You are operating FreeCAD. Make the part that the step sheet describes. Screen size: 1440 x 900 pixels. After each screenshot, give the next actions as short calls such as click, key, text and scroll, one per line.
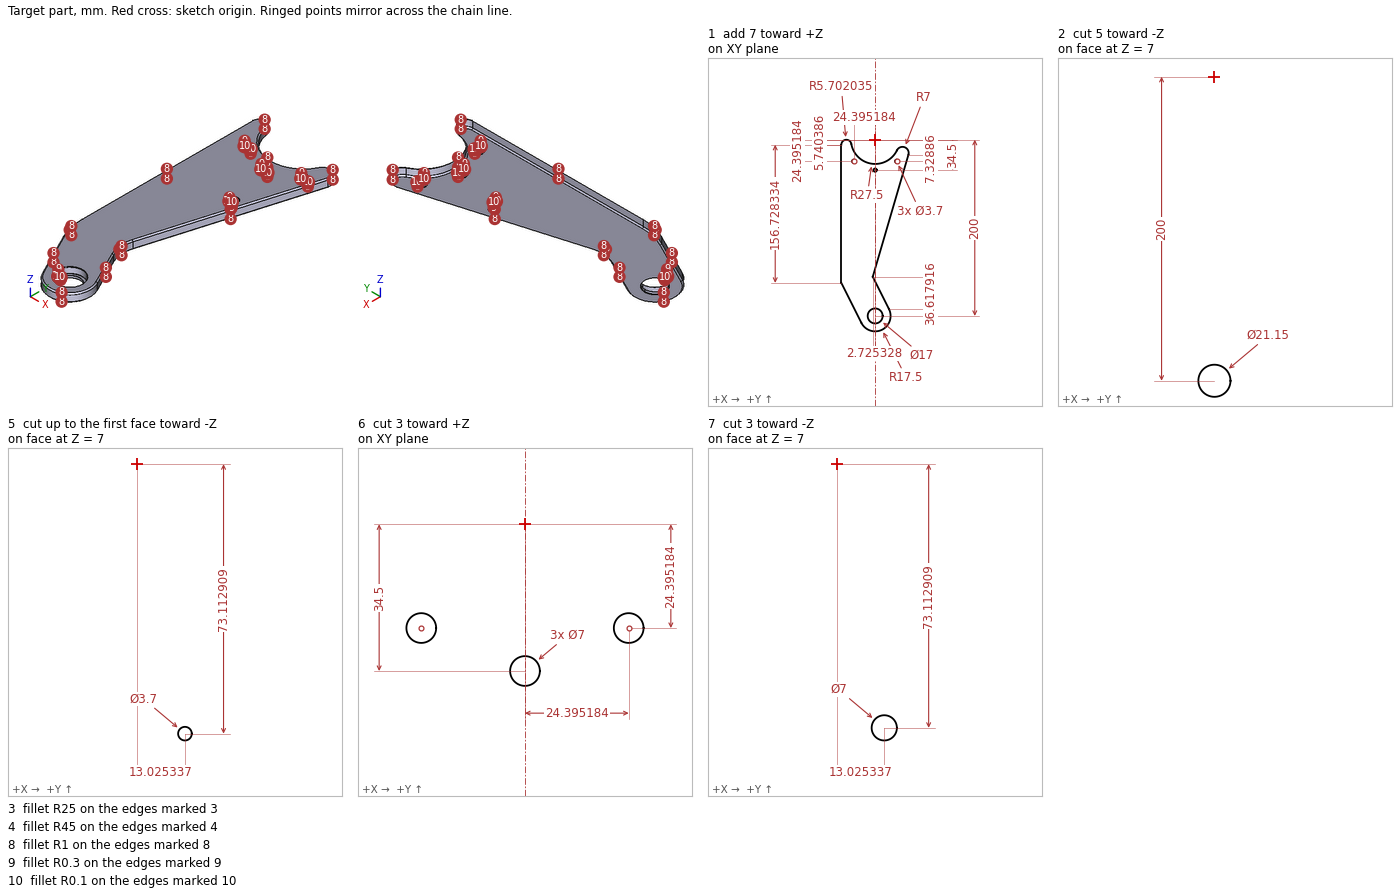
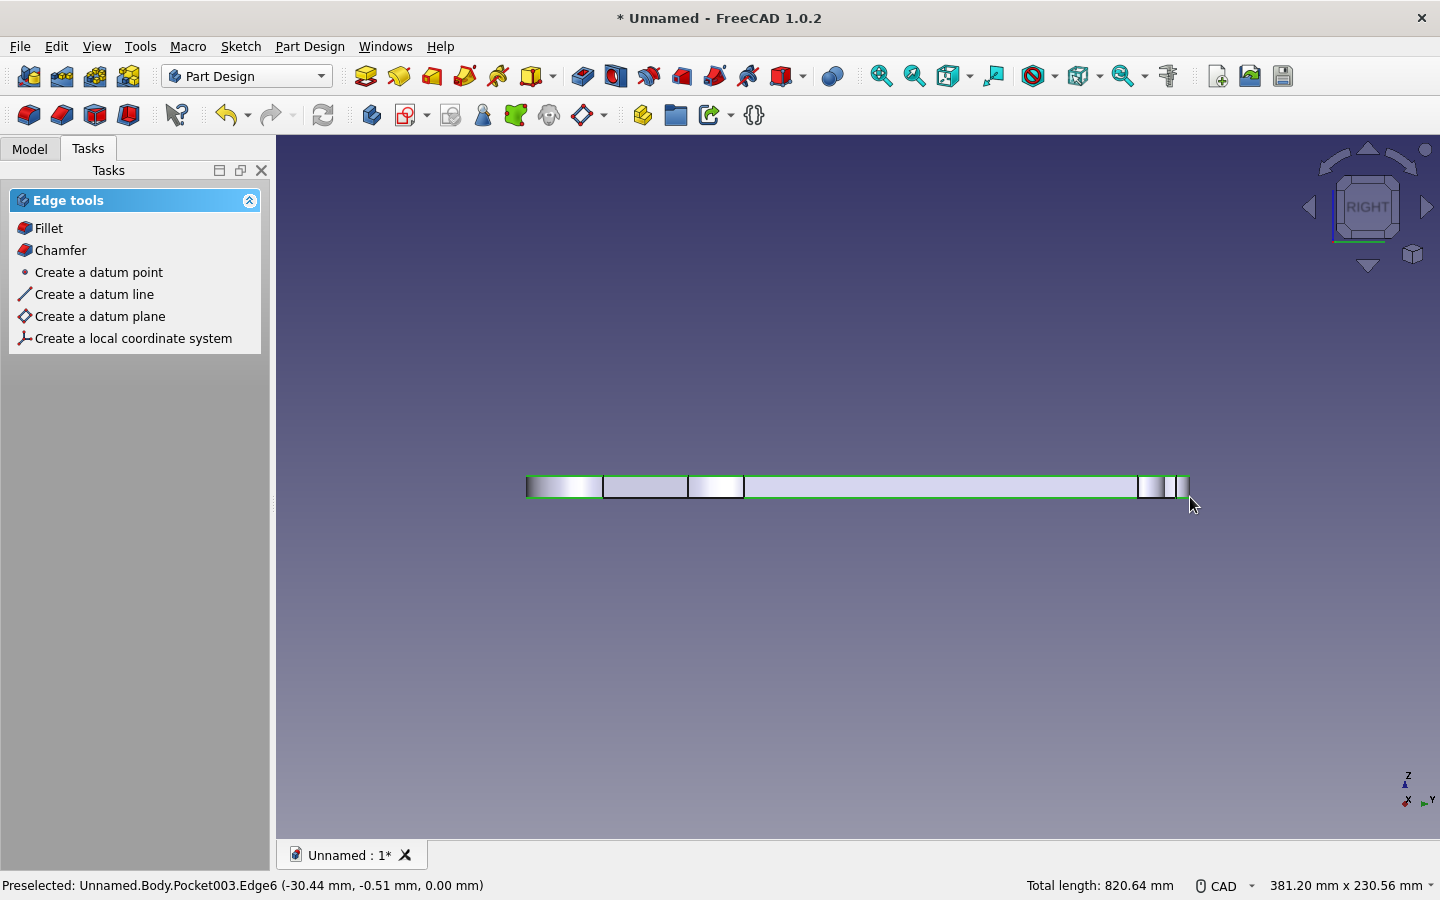
click(1169, 497, ctrl)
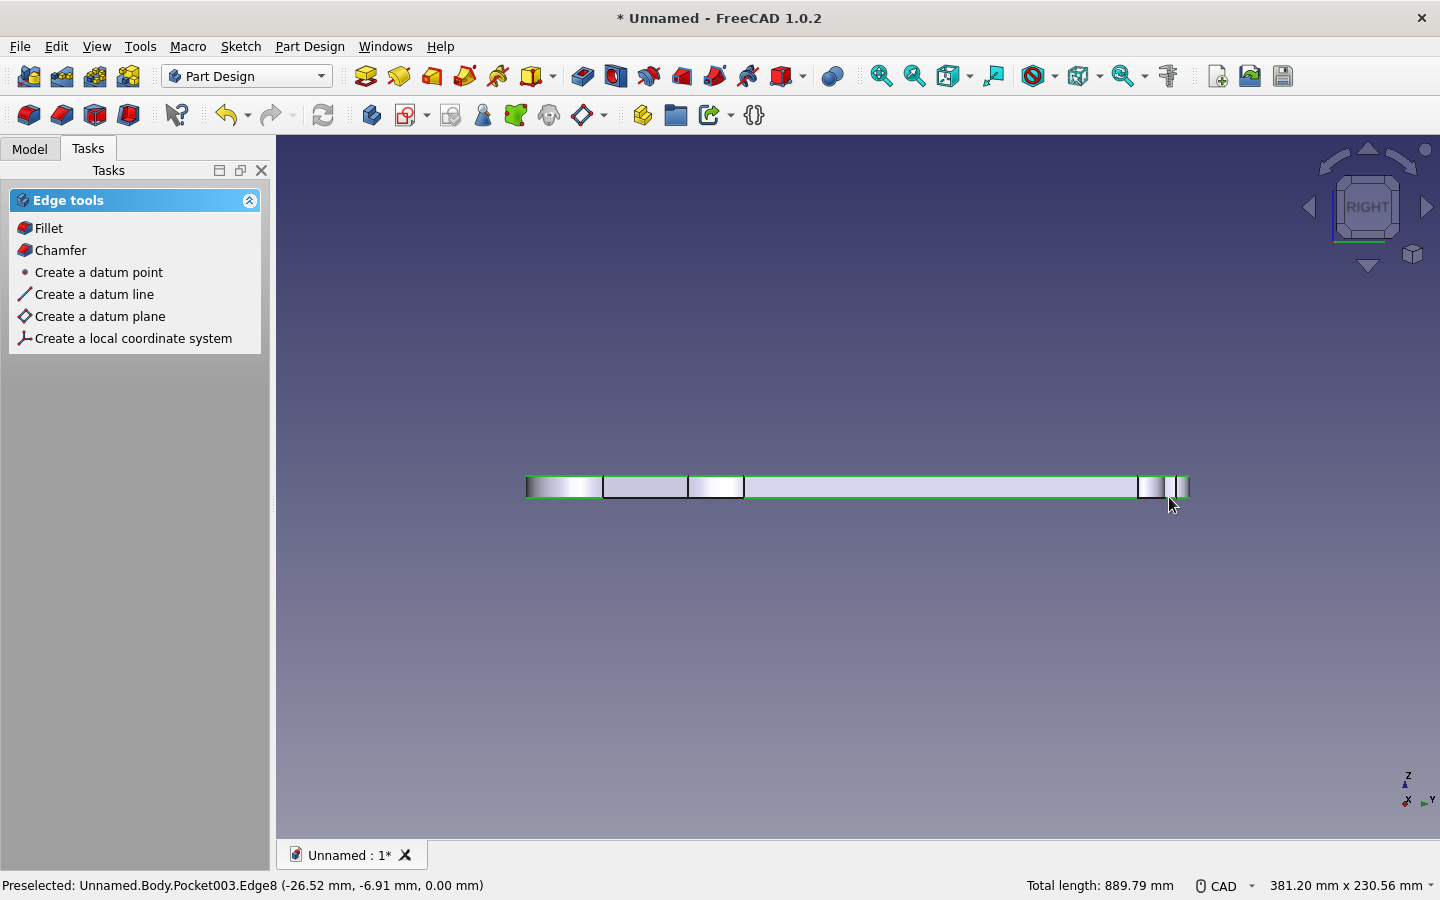
click(1164, 497, ctrl)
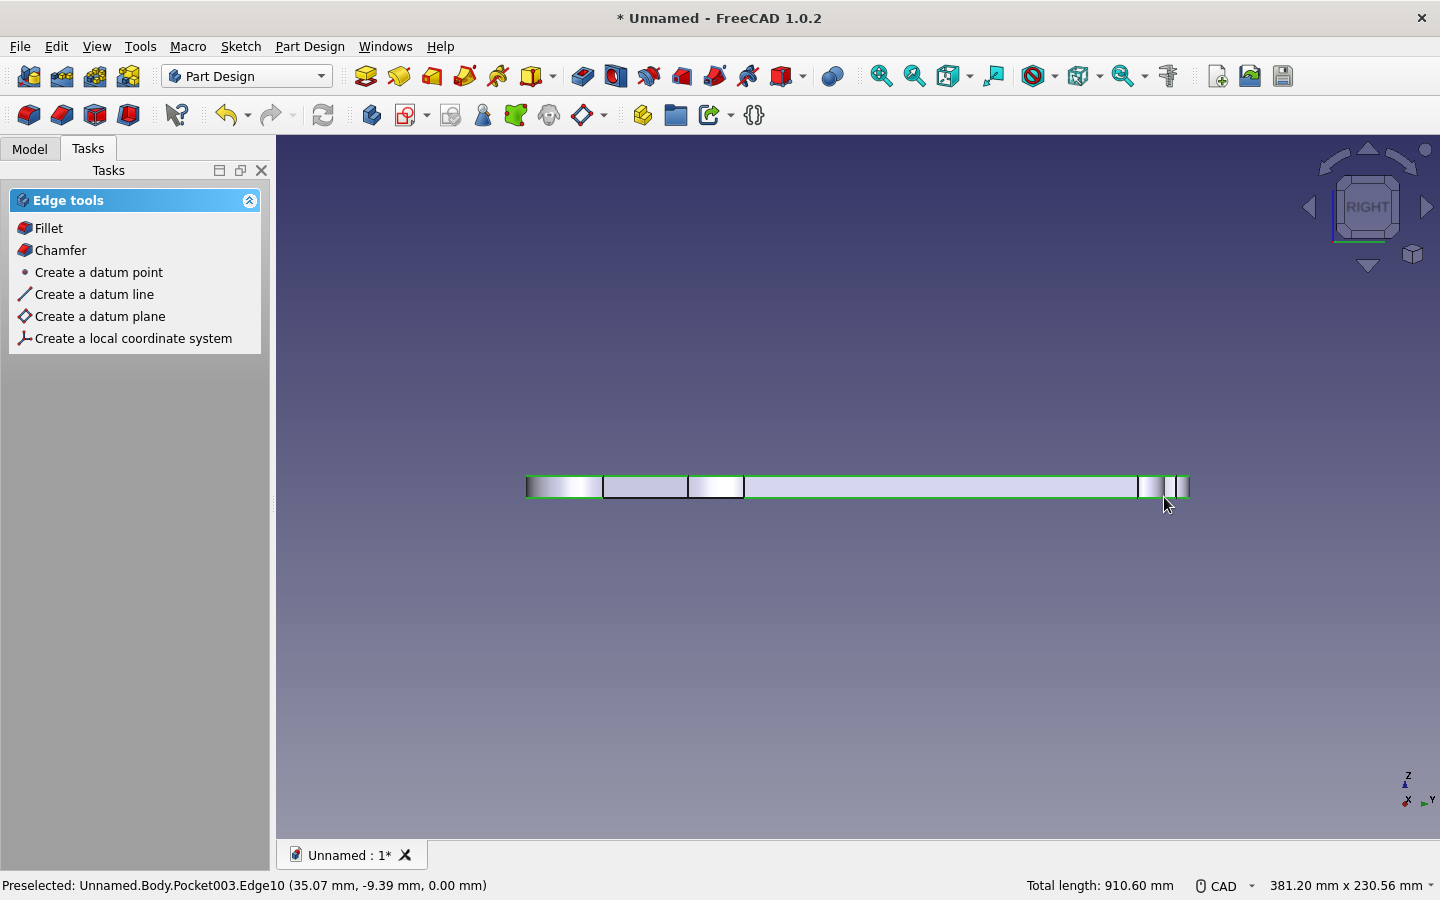
click(646, 497, ctrl)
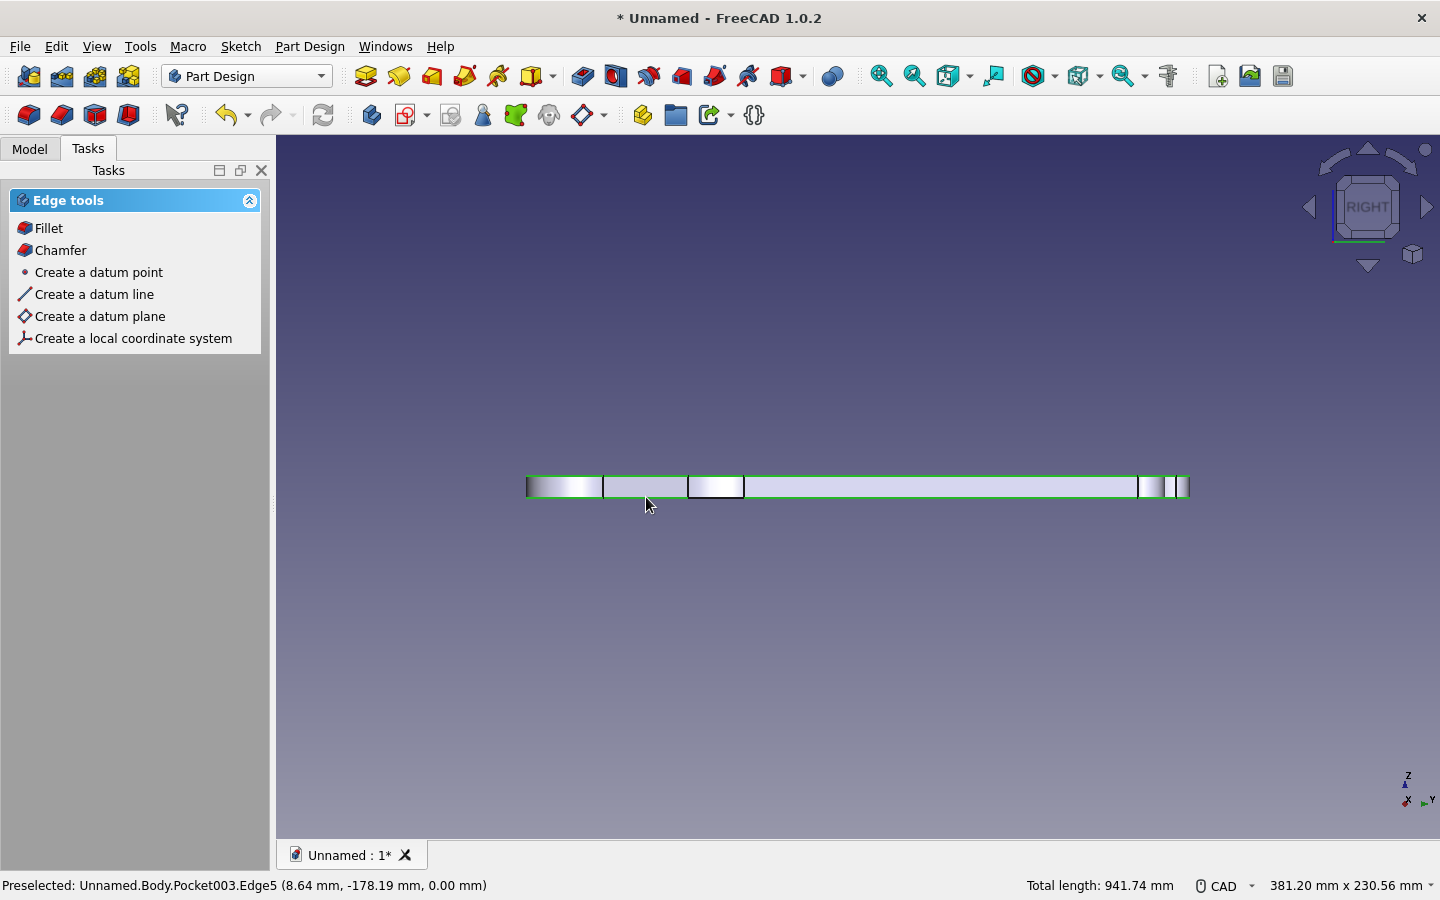
click(716, 497, ctrl)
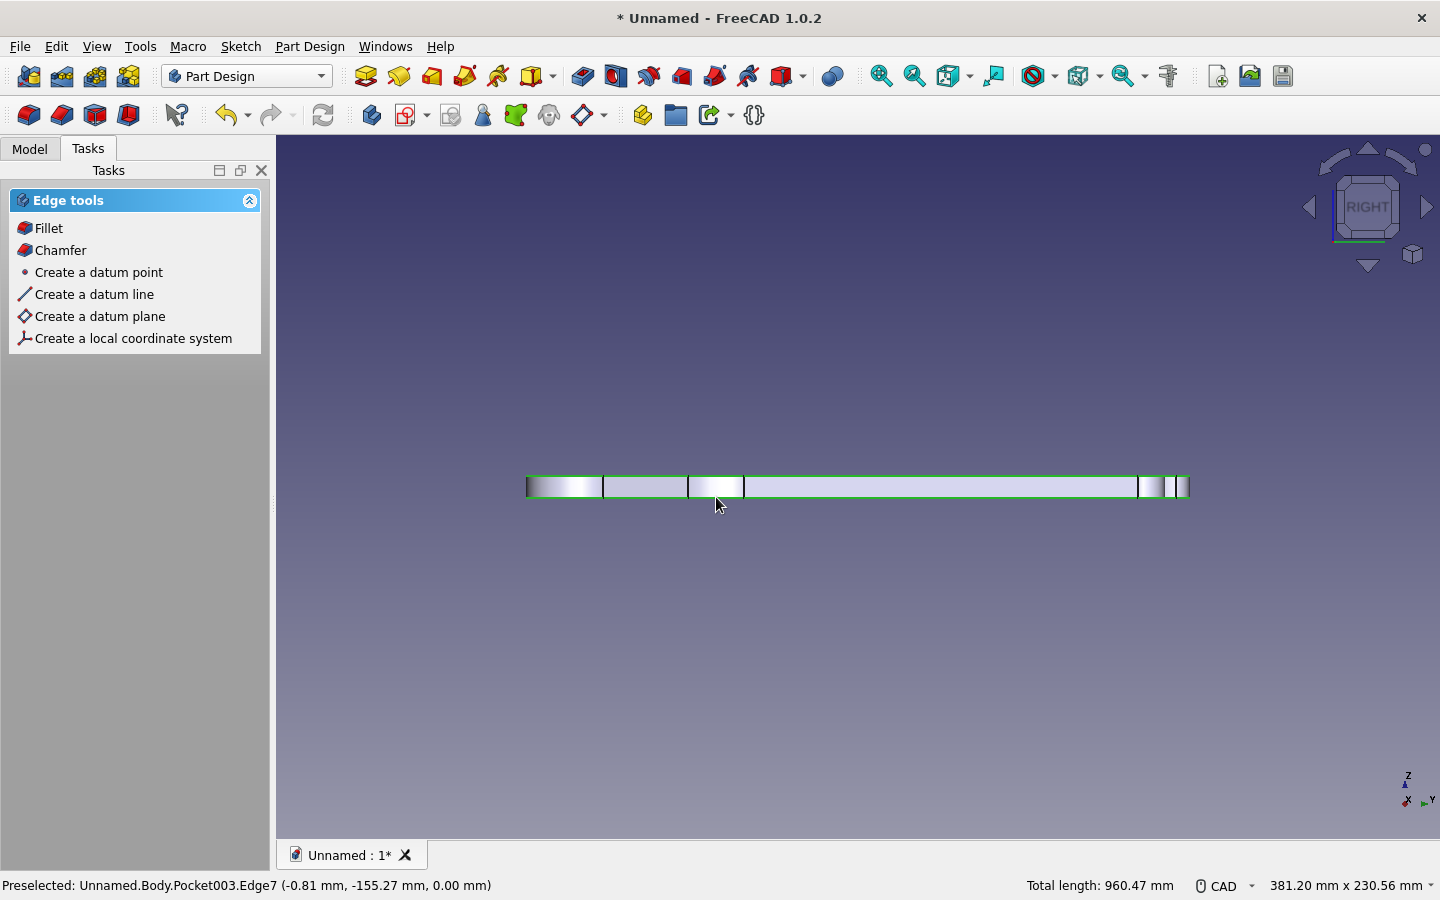
key(5)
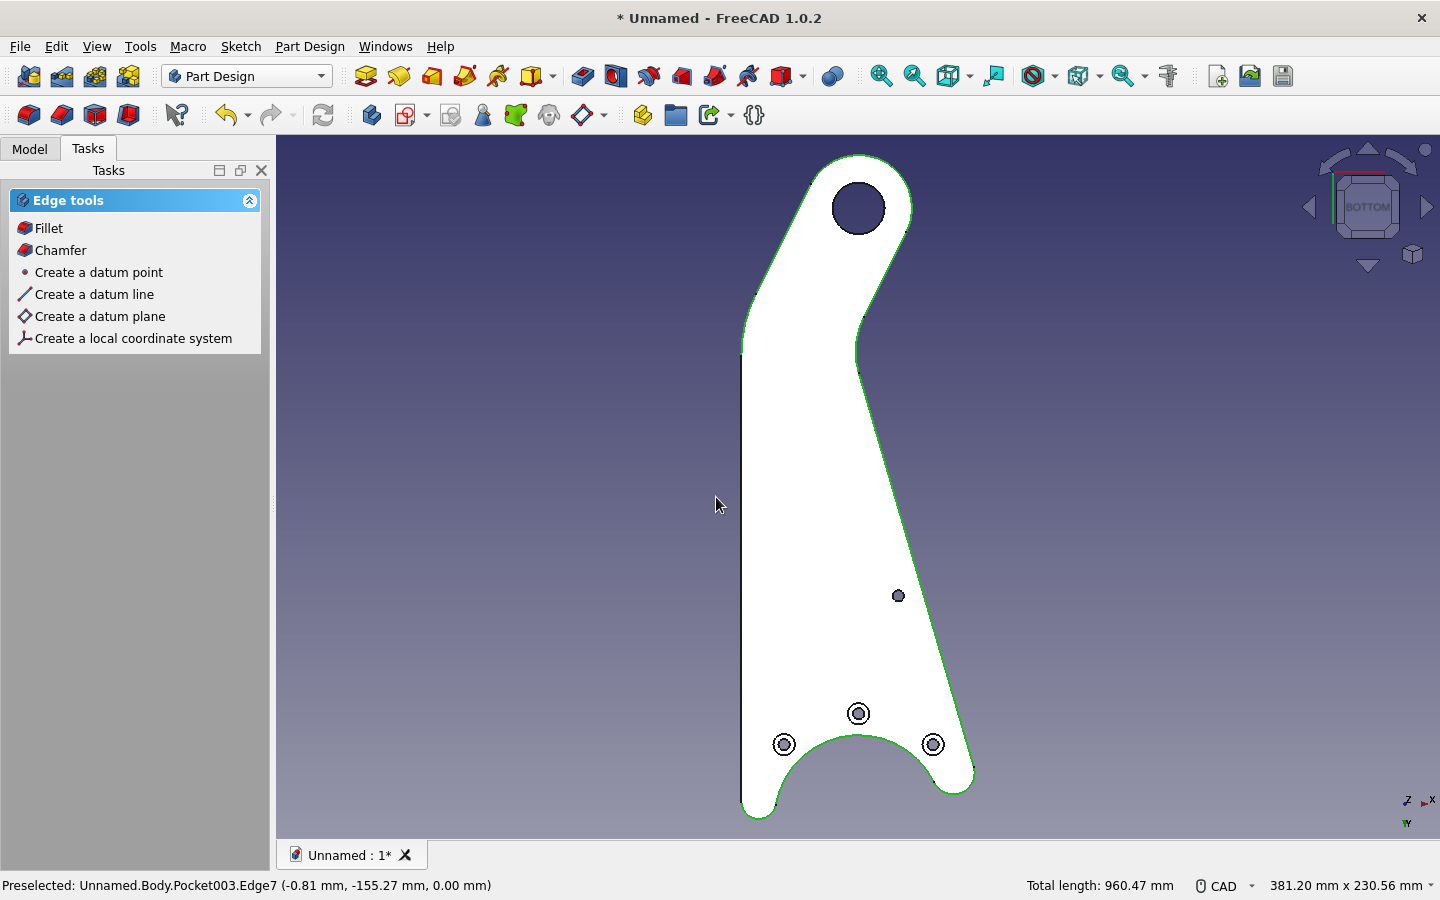
click(741, 578, ctrl)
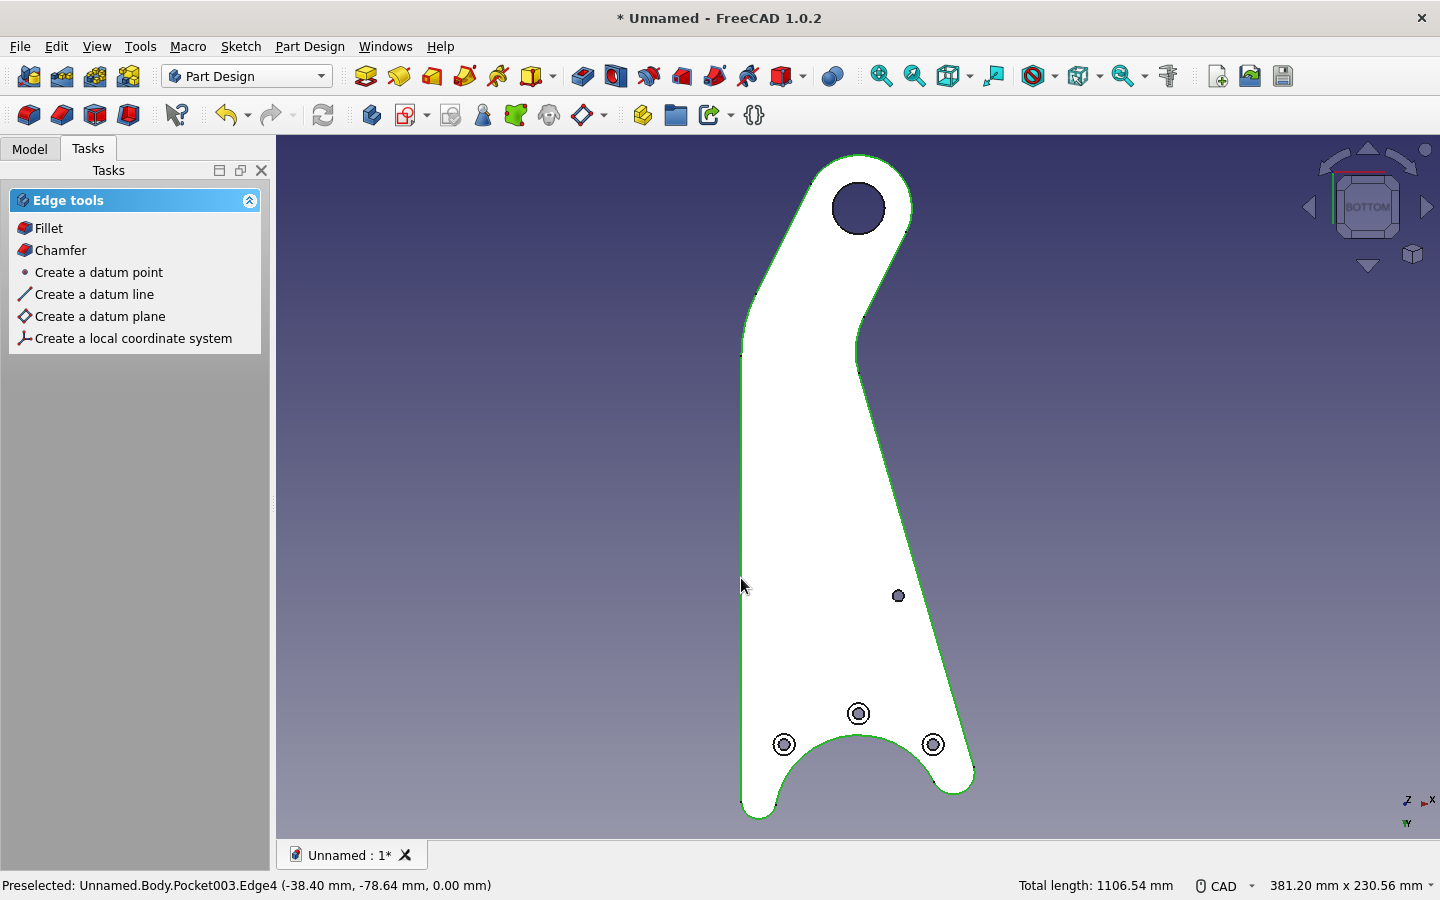
click(29, 116)